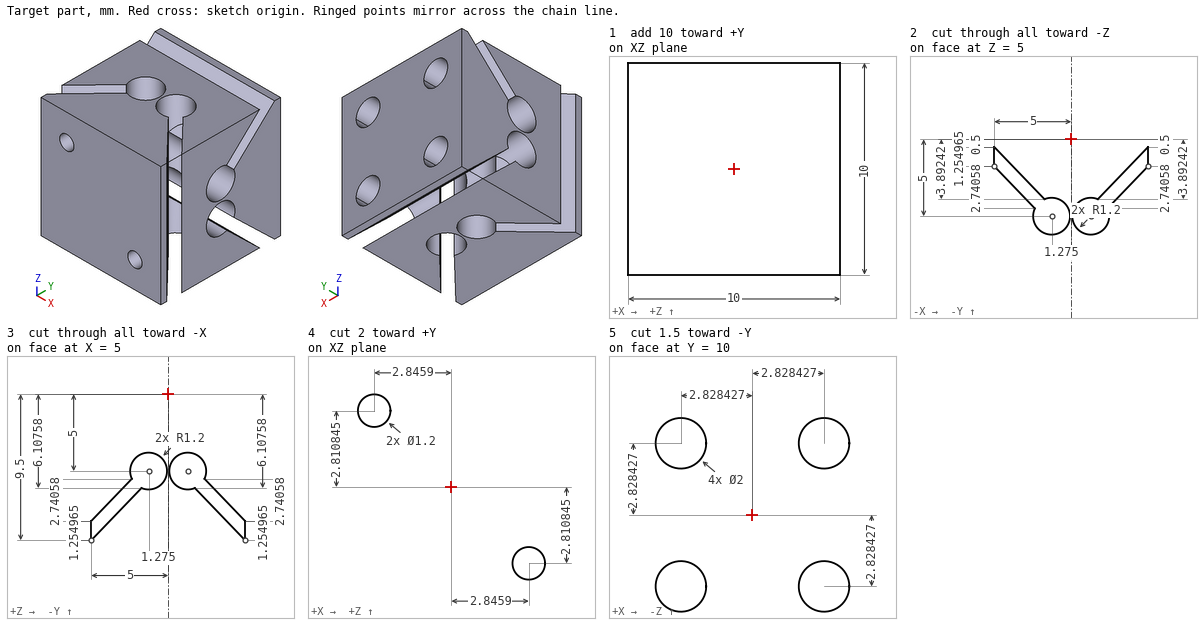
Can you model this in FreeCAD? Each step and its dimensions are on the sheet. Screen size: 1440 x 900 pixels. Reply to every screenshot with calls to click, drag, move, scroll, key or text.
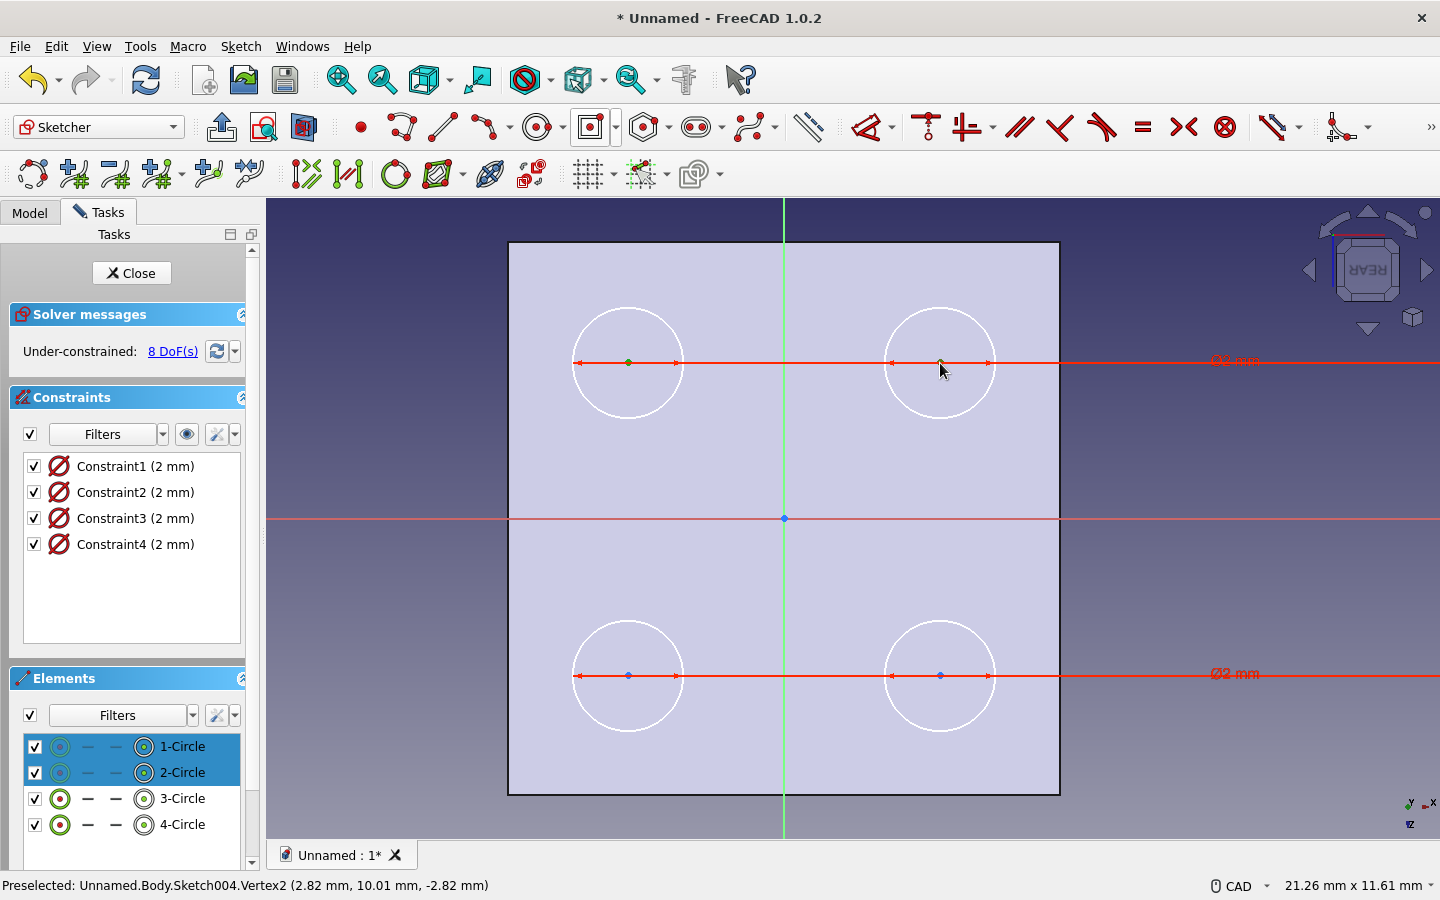
click(992, 128)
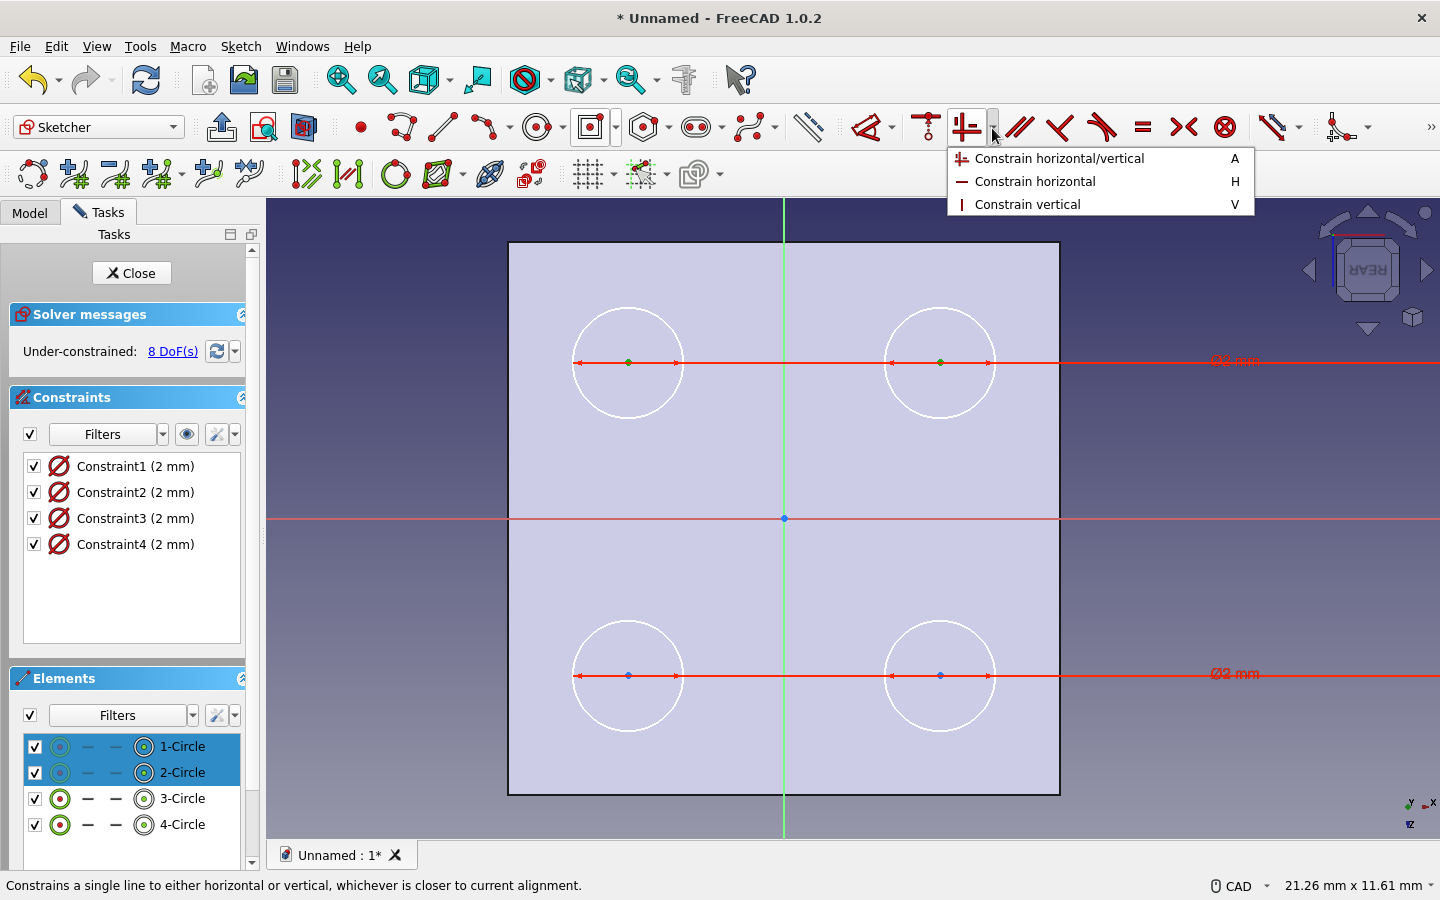
click(1101, 182)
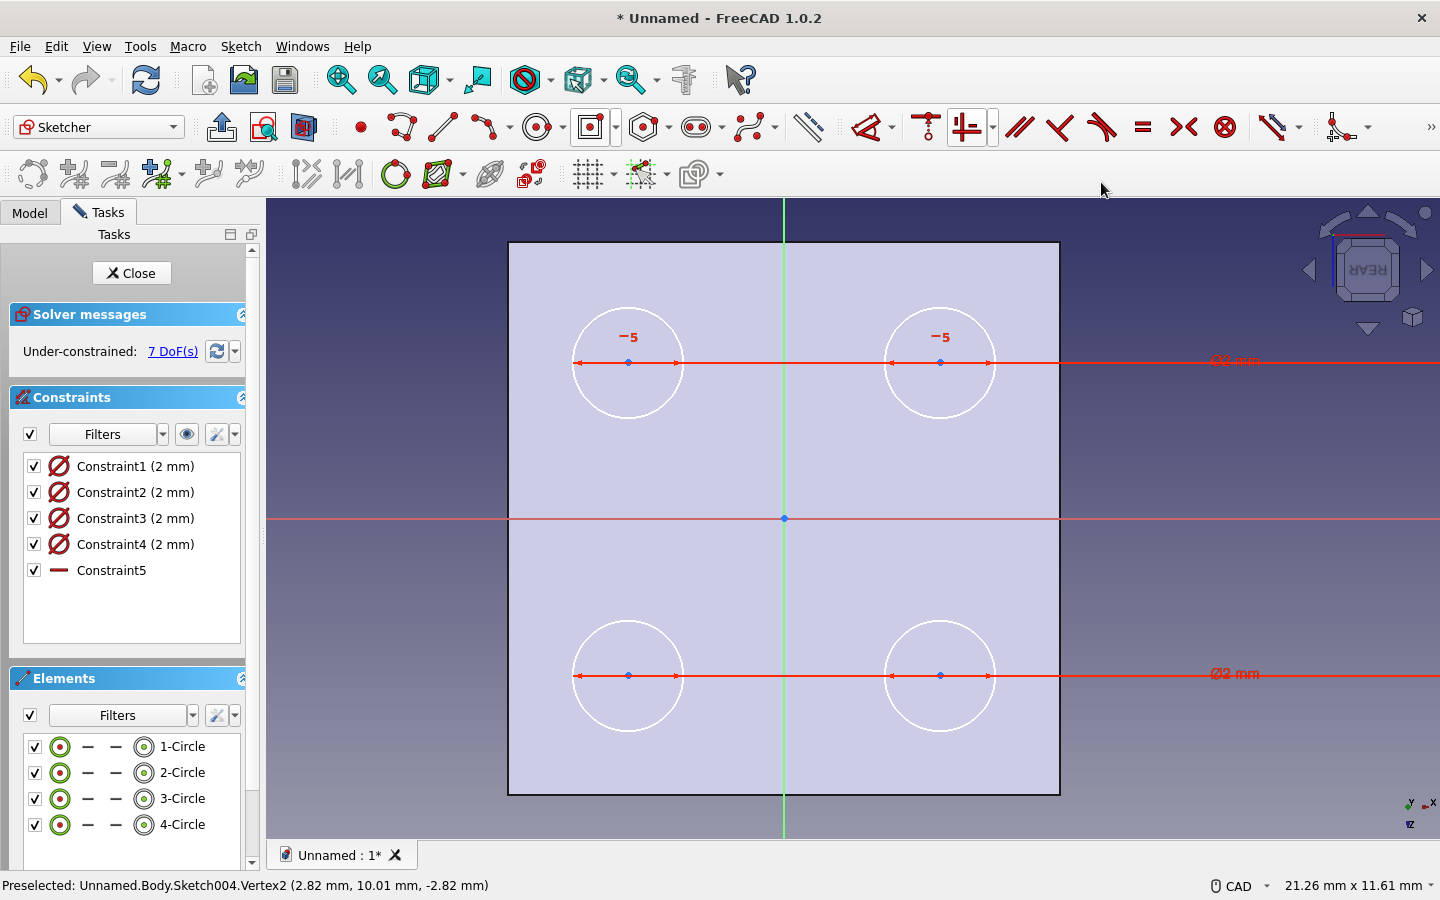
click(940, 363)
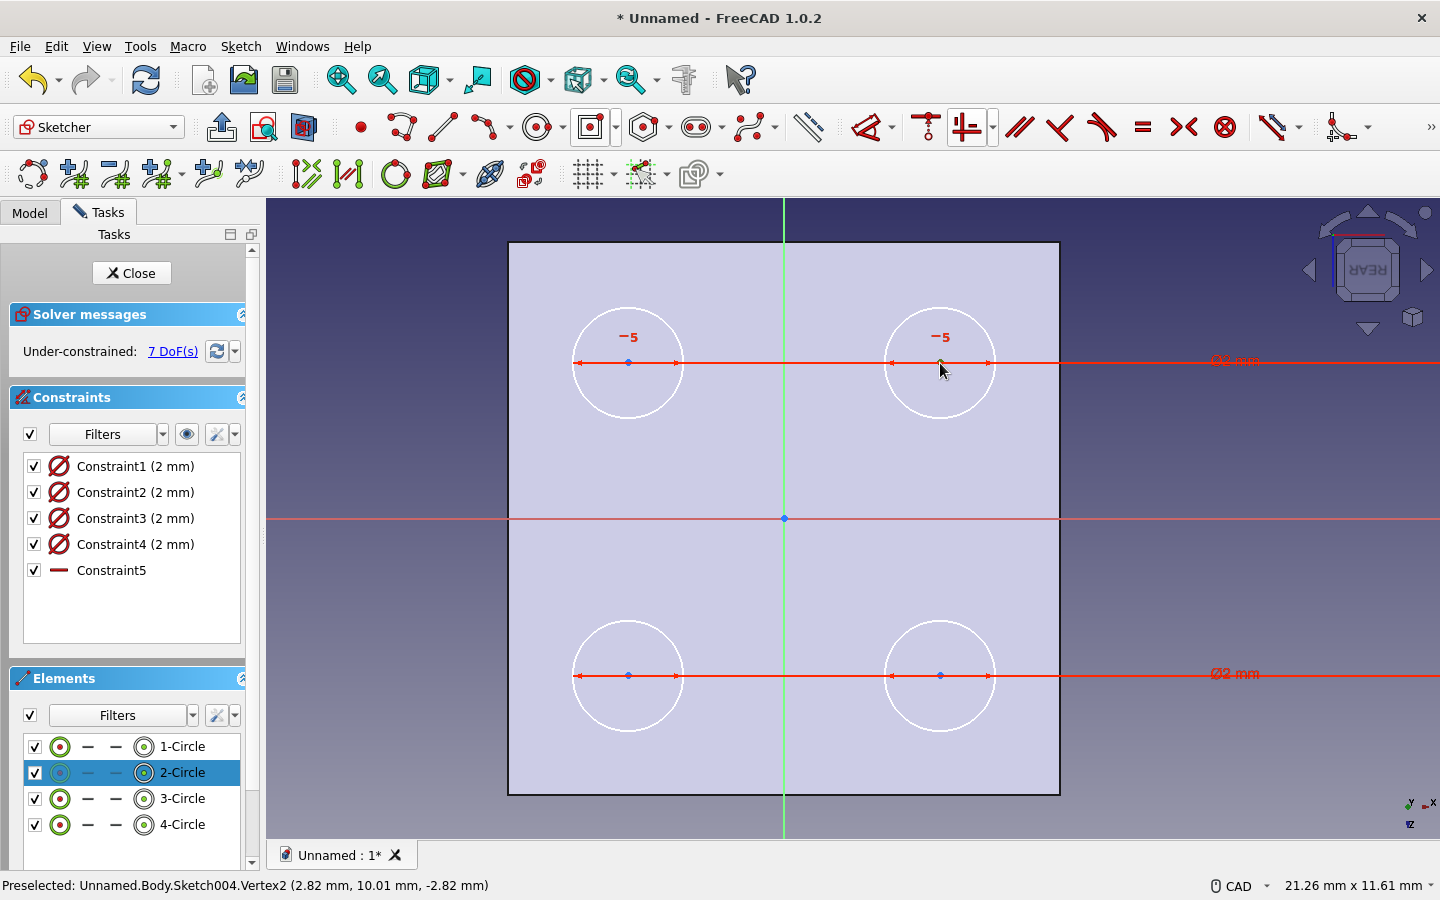
click(940, 676)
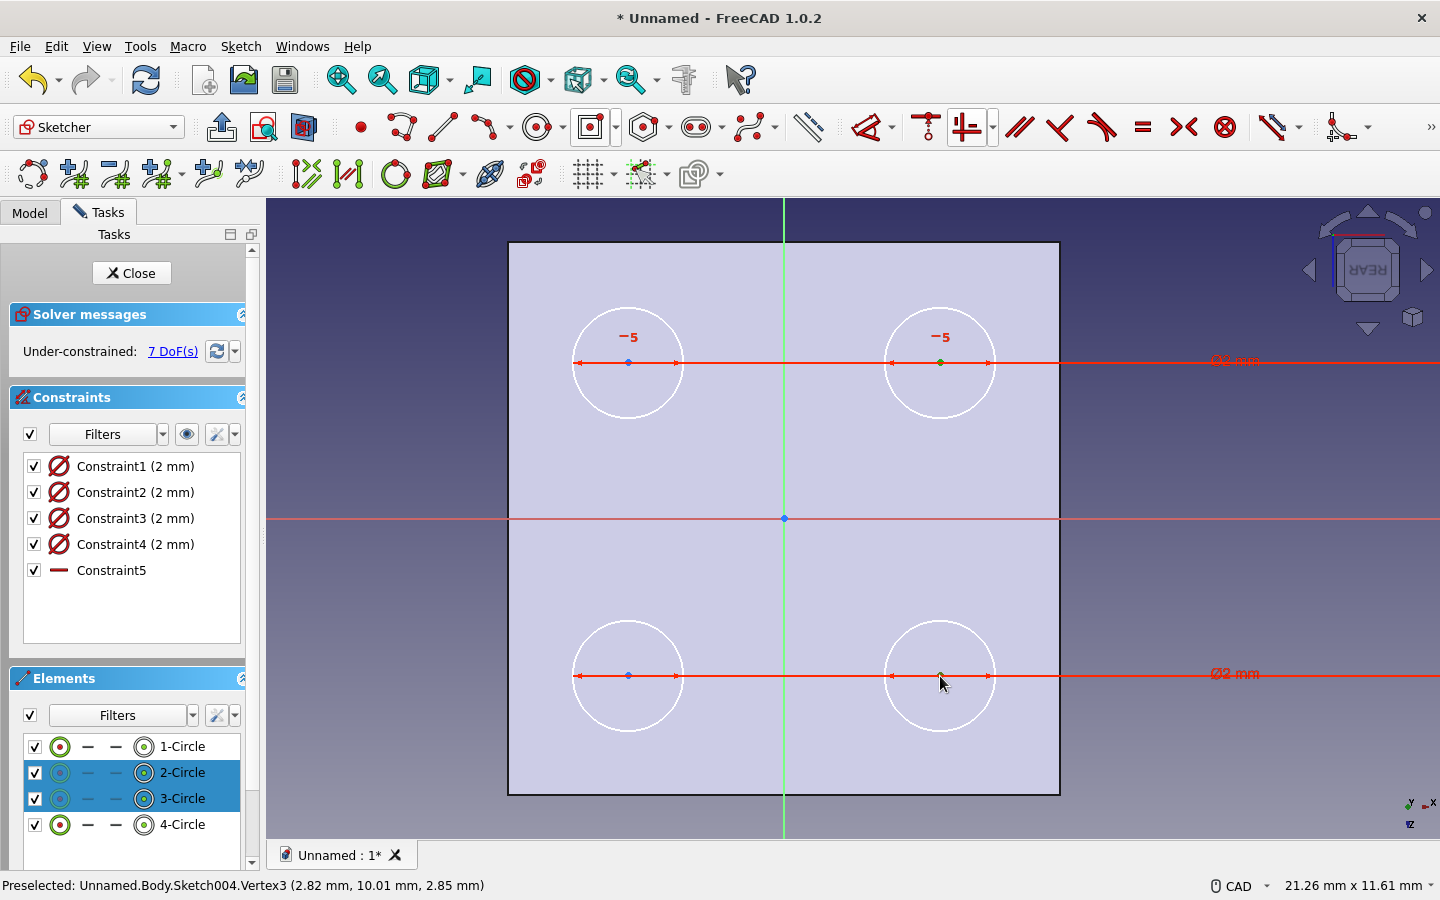
click(992, 128)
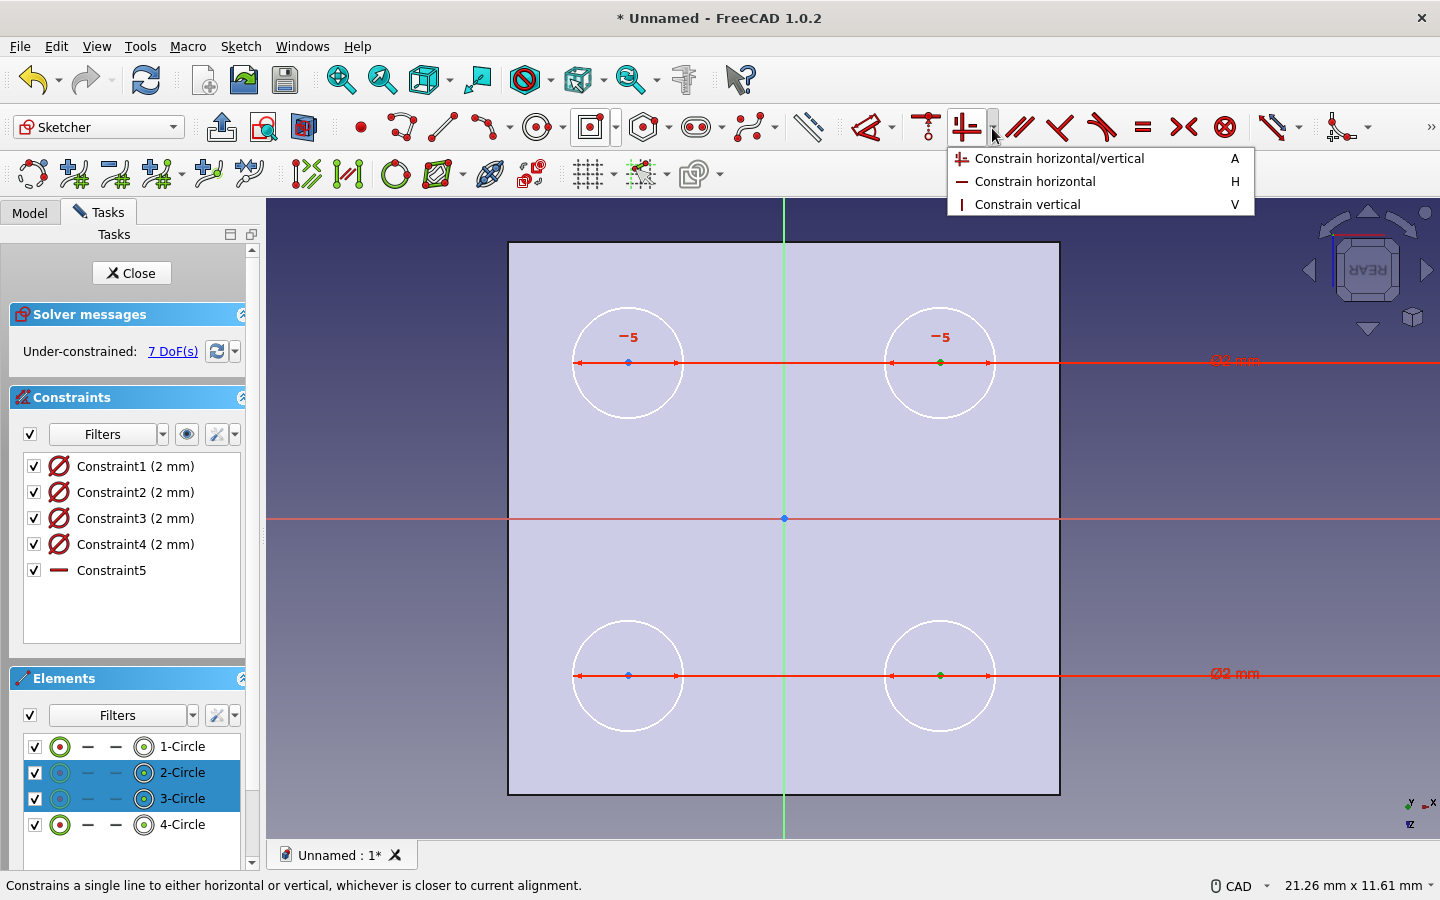
click(1101, 204)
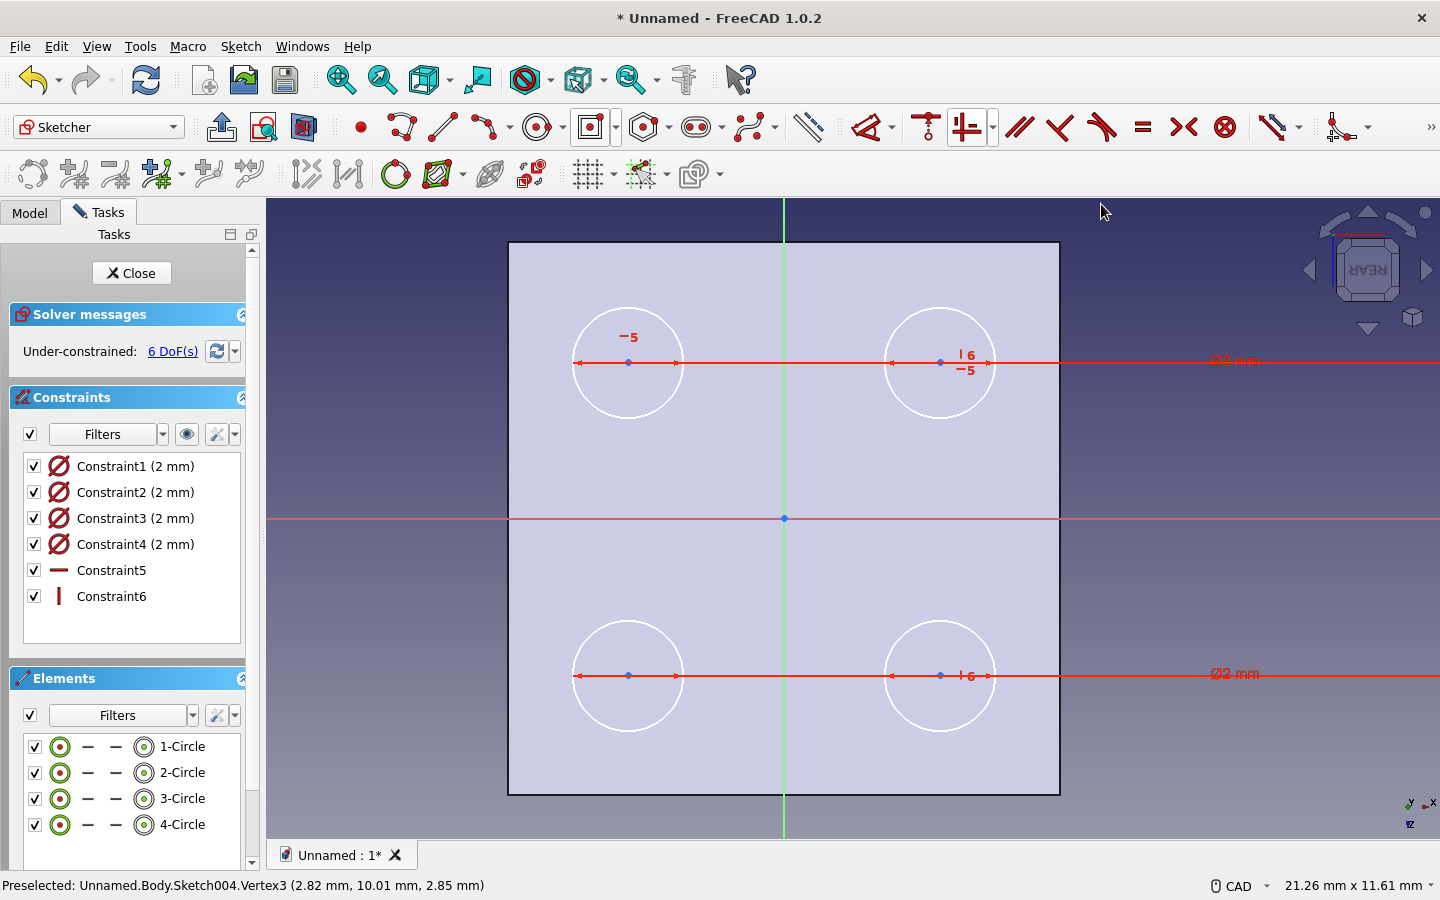
click(628, 363)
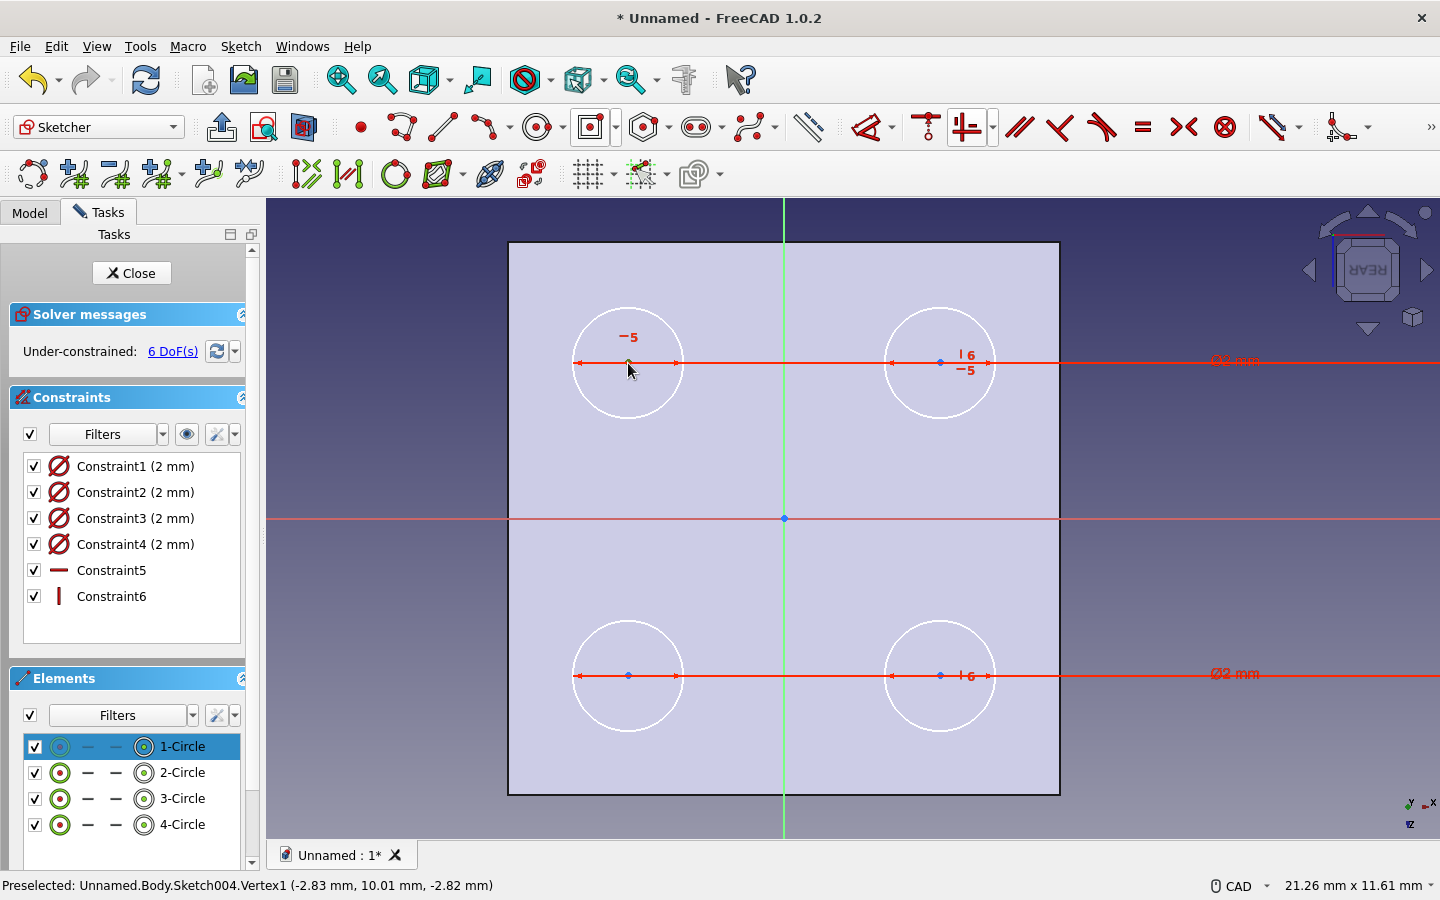
click(628, 676)